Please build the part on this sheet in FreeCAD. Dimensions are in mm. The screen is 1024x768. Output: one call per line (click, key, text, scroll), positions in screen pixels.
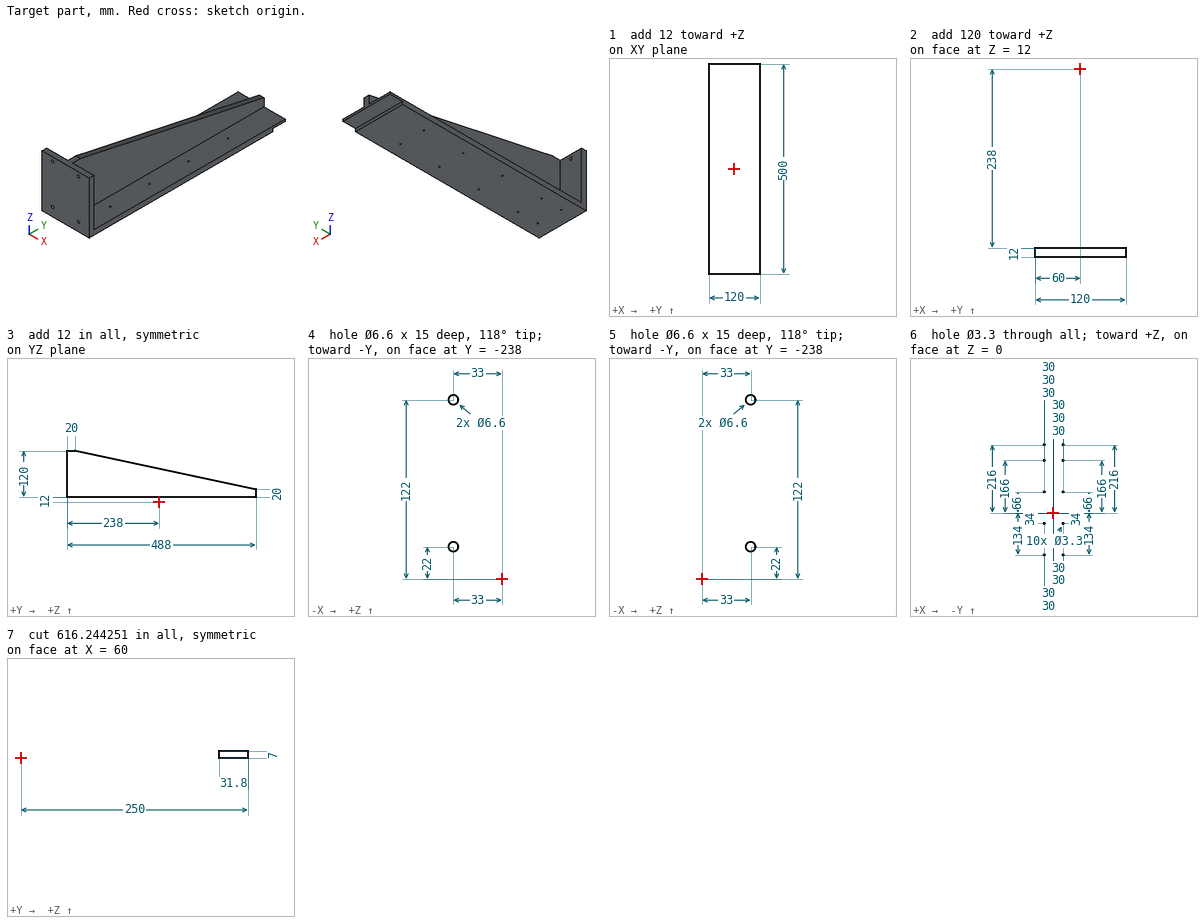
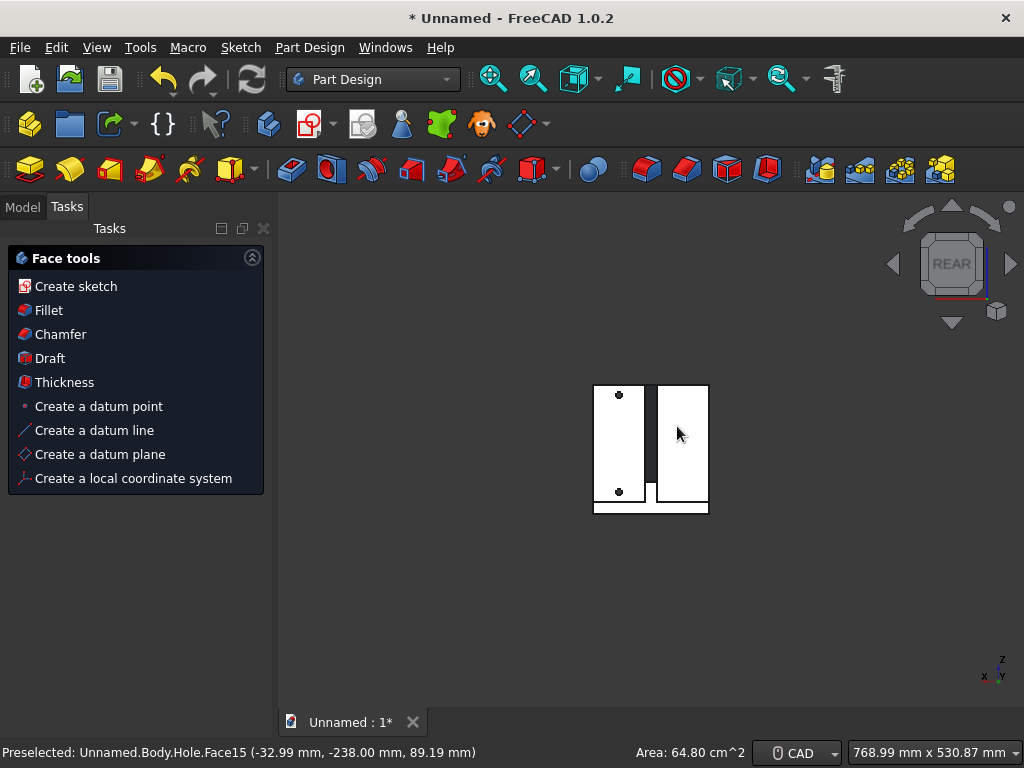
click(310, 124)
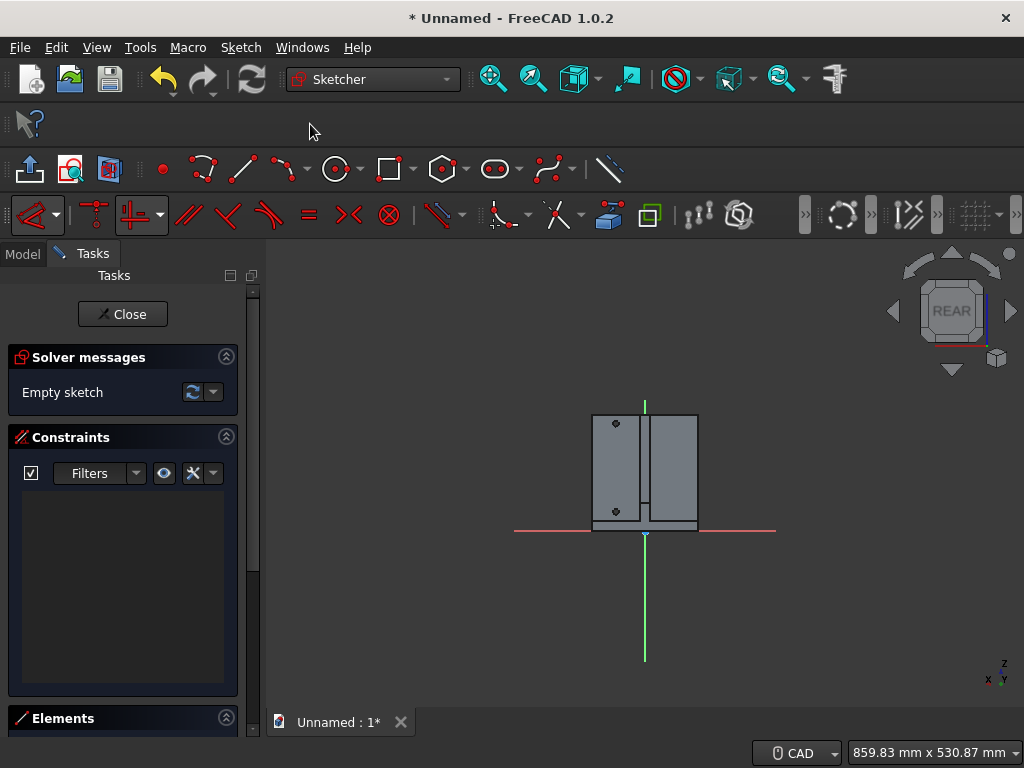
click(110, 170)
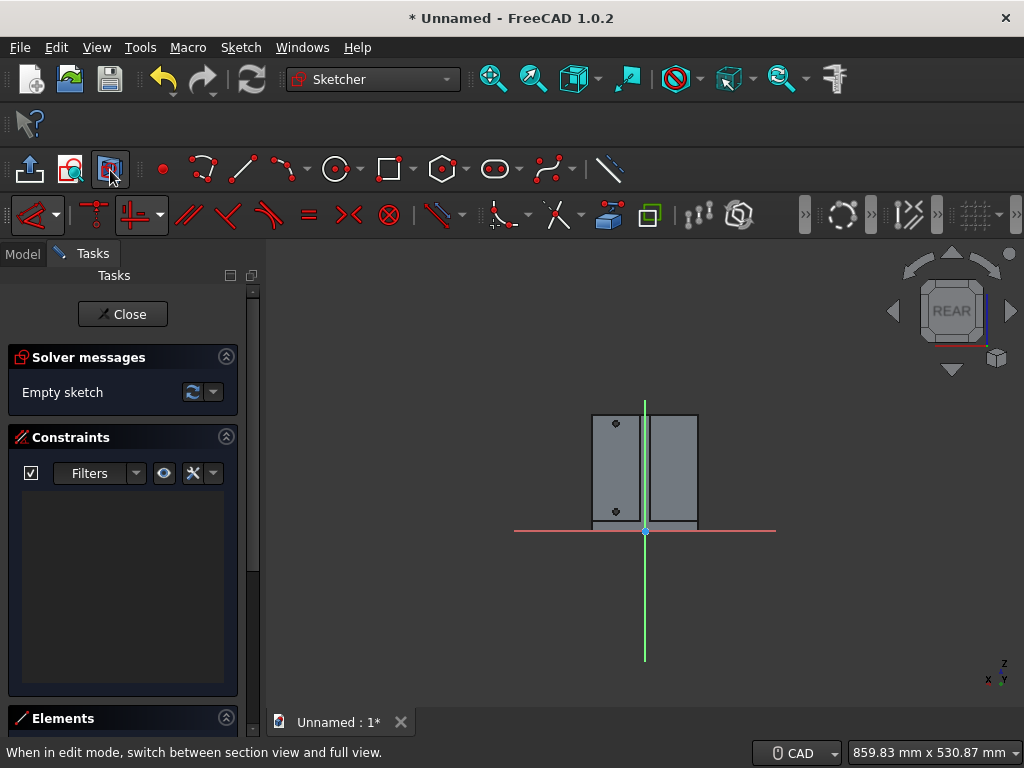
scroll(710, 478, up, 5)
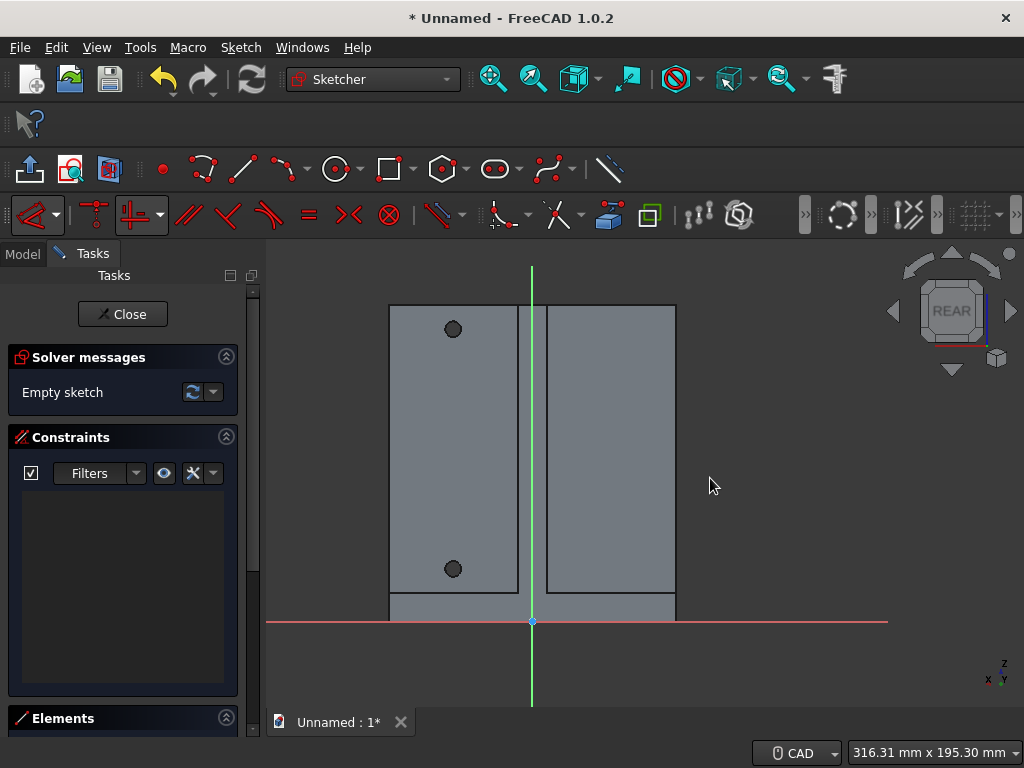
click(336, 170)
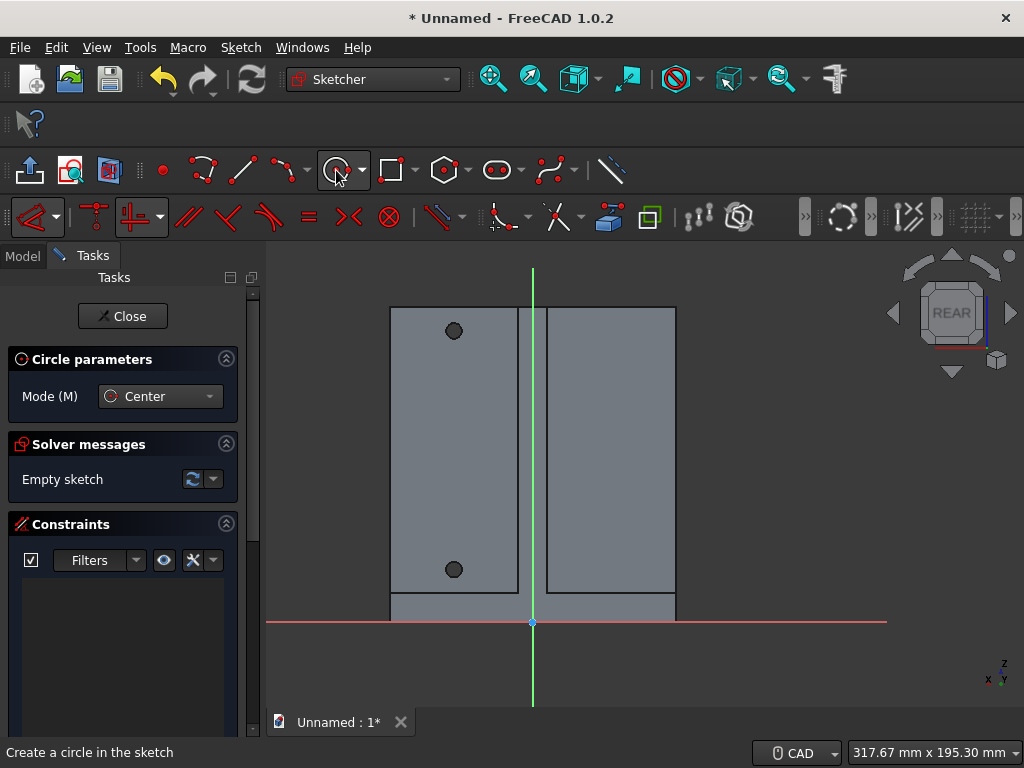
scroll(612, 331, up, 6)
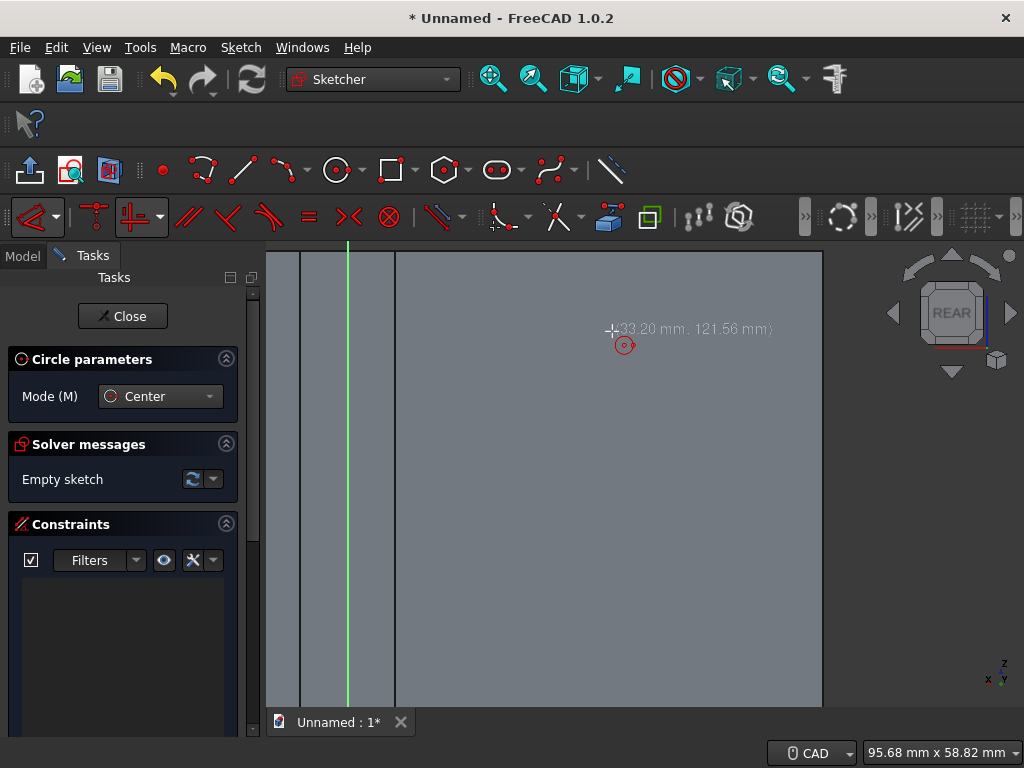
click(609, 330)
click(628, 312)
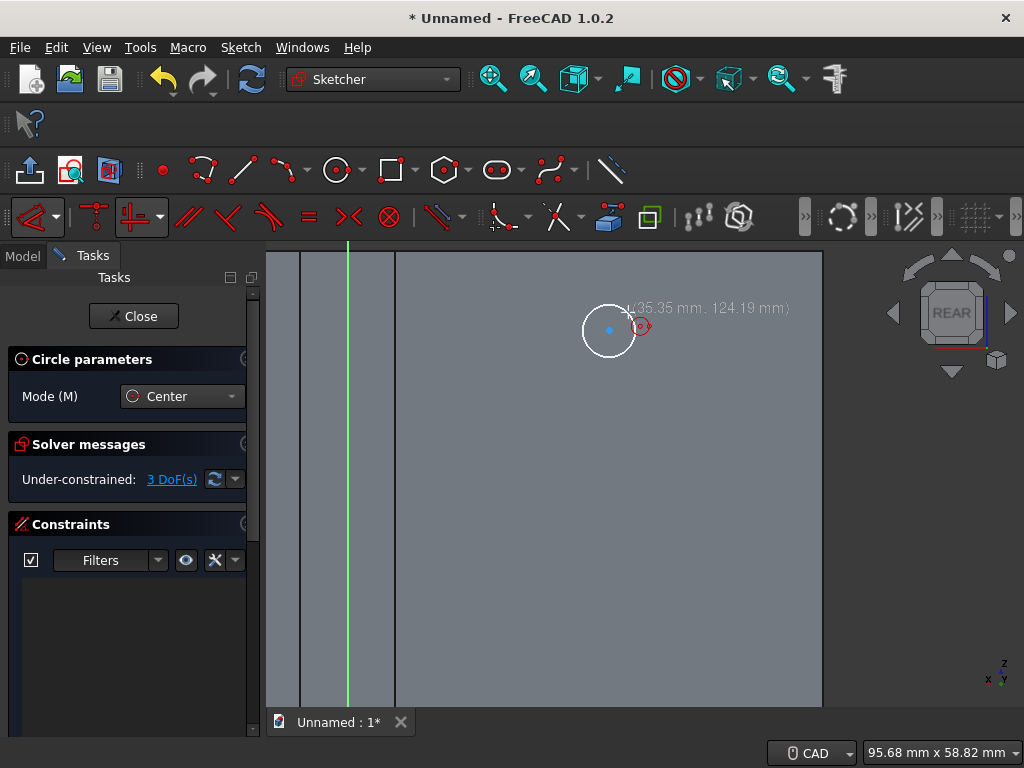
scroll(613, 333, down, 6)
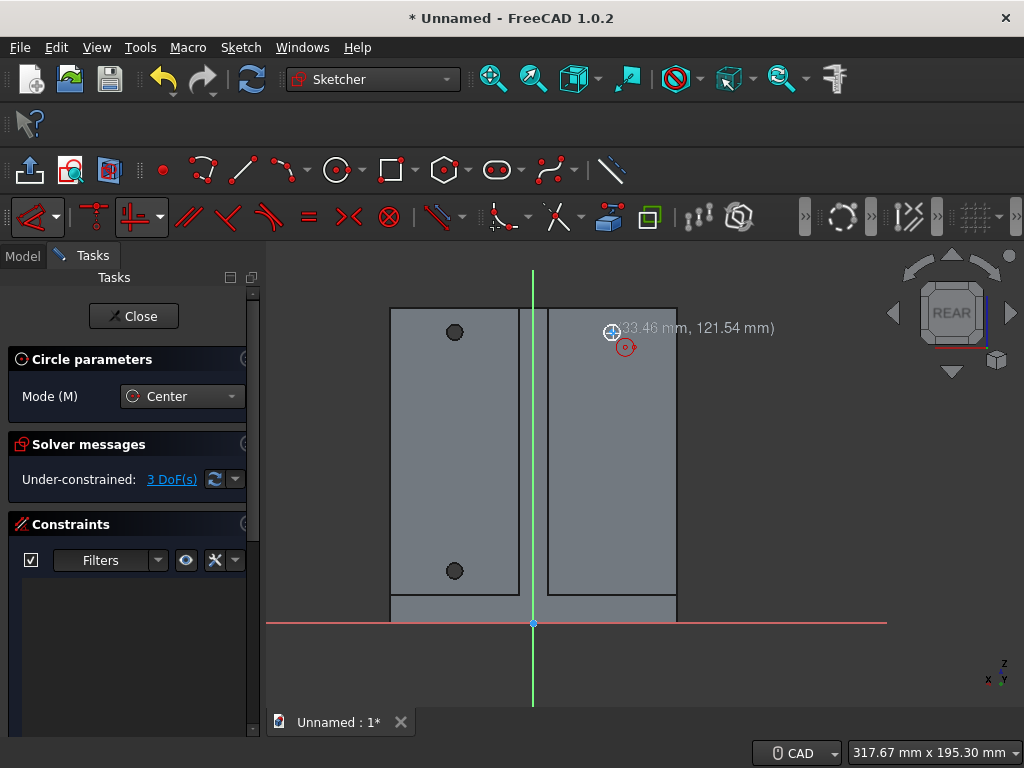
scroll(612, 571, up, 6)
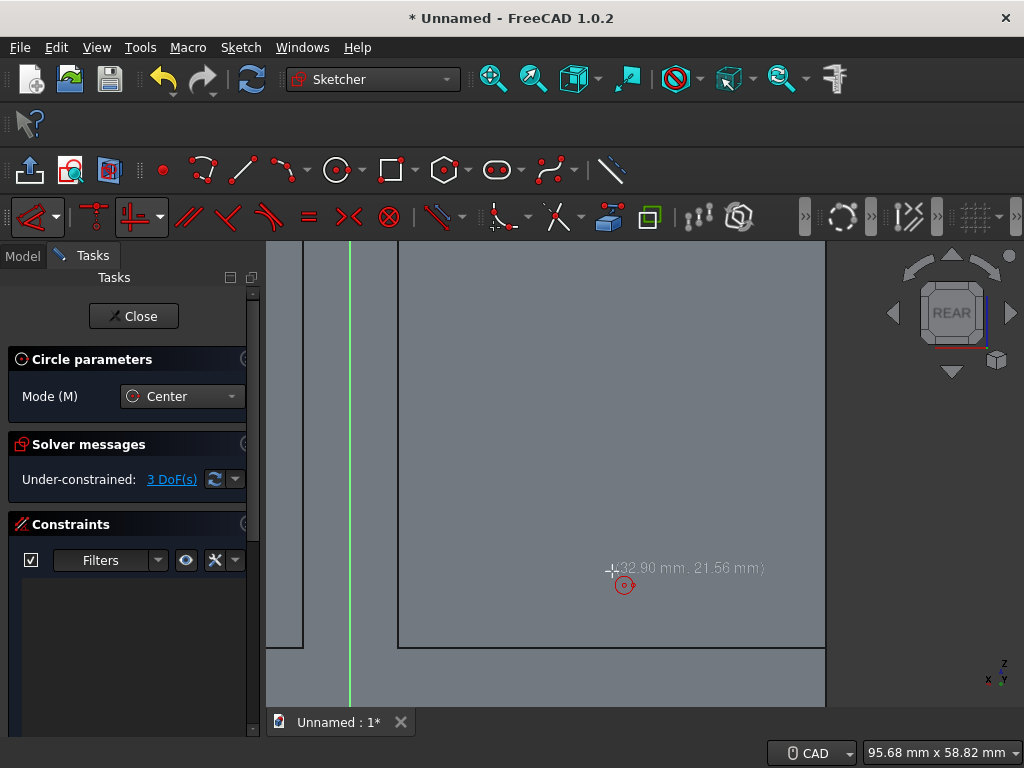
click(612, 569)
click(630, 551)
key(Escape)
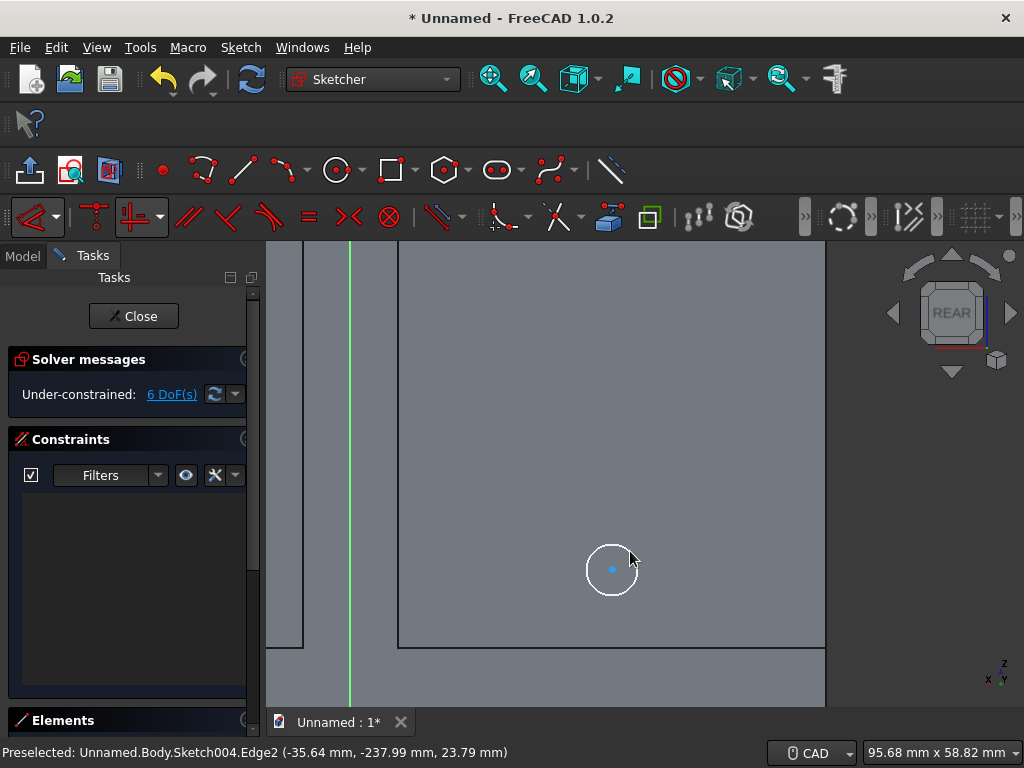
scroll(612, 572, down, 6)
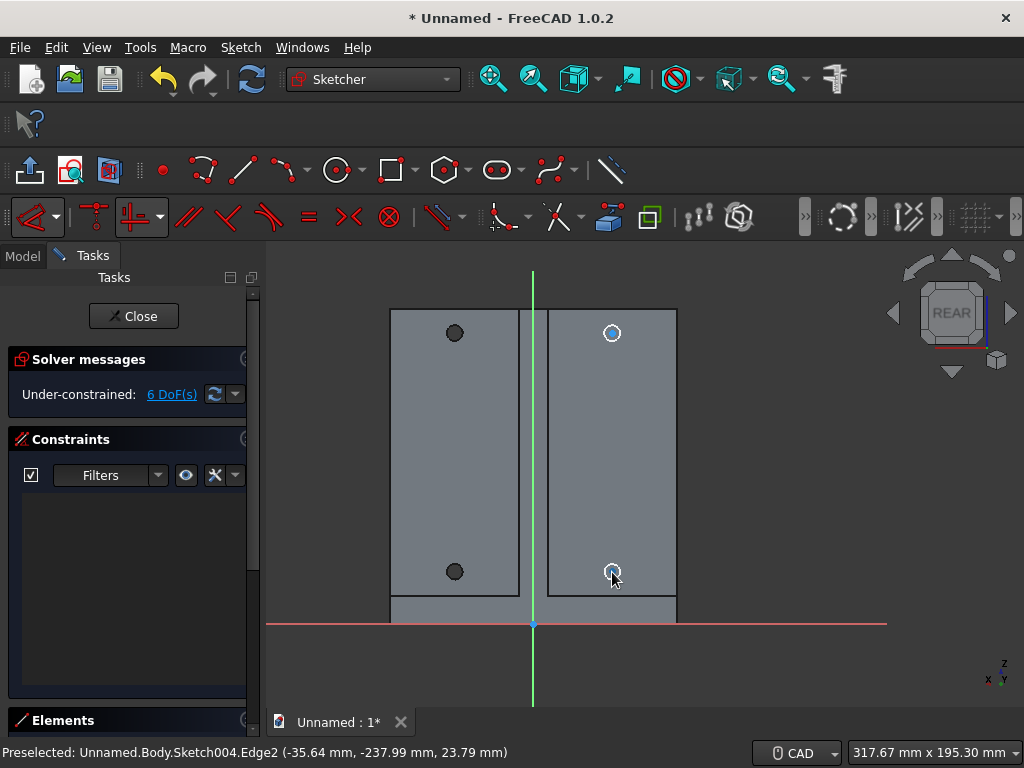
scroll(618, 328, up, 3)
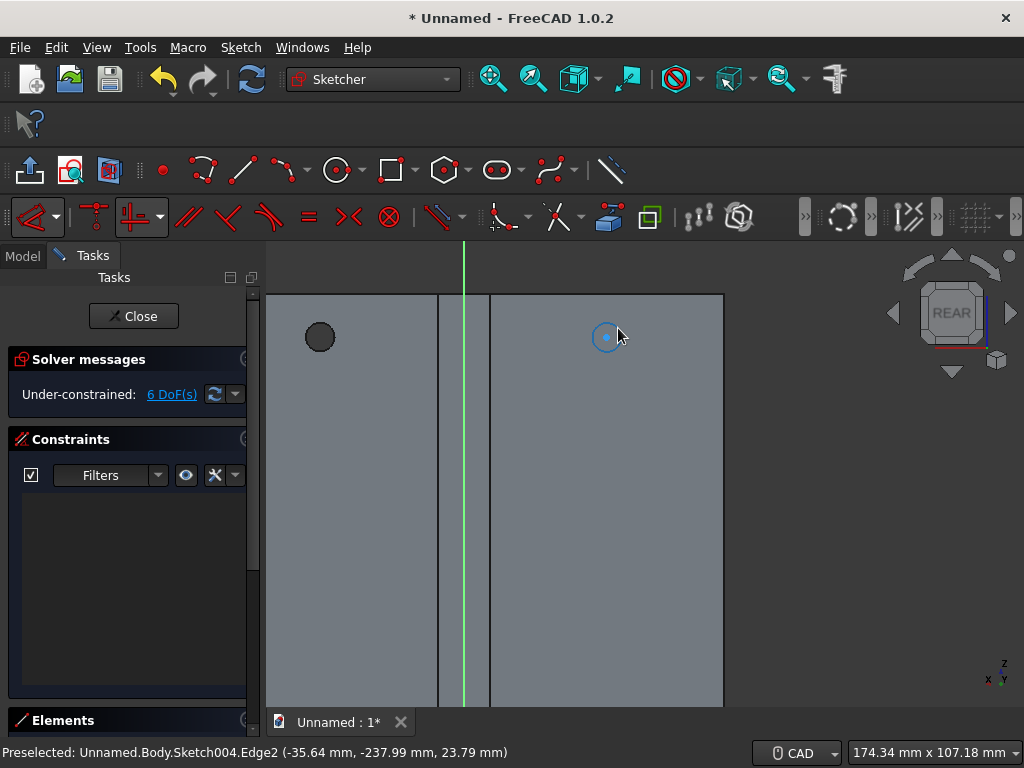
click(617, 327)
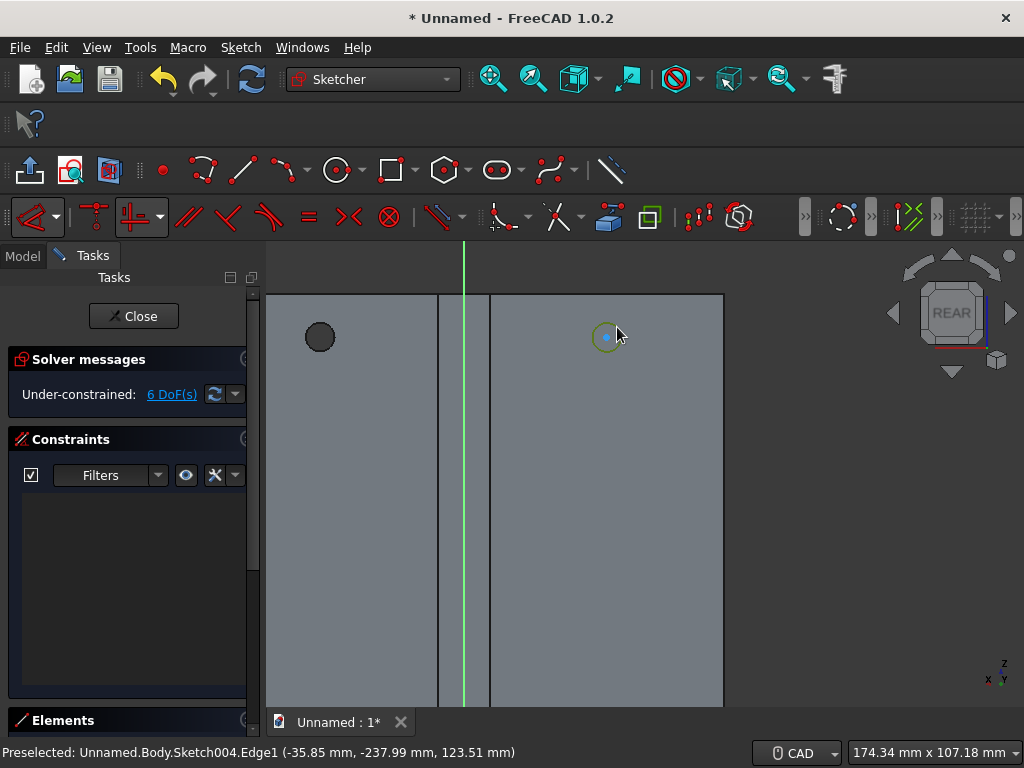
scroll(618, 327, down, 3)